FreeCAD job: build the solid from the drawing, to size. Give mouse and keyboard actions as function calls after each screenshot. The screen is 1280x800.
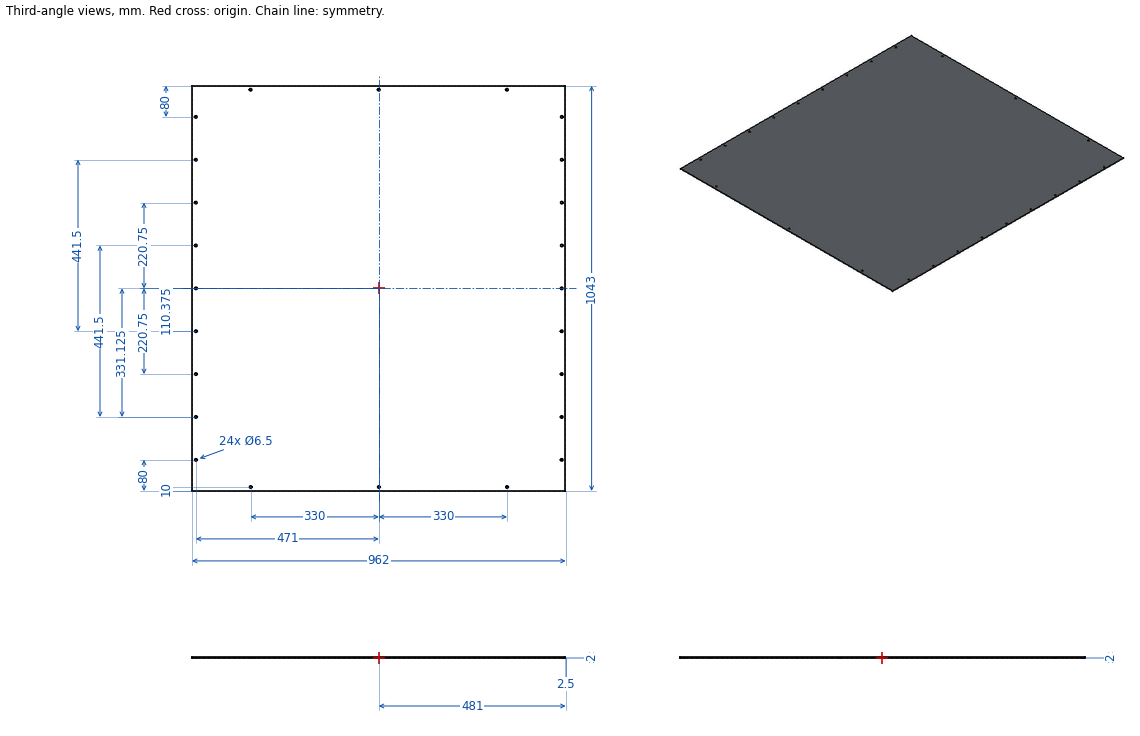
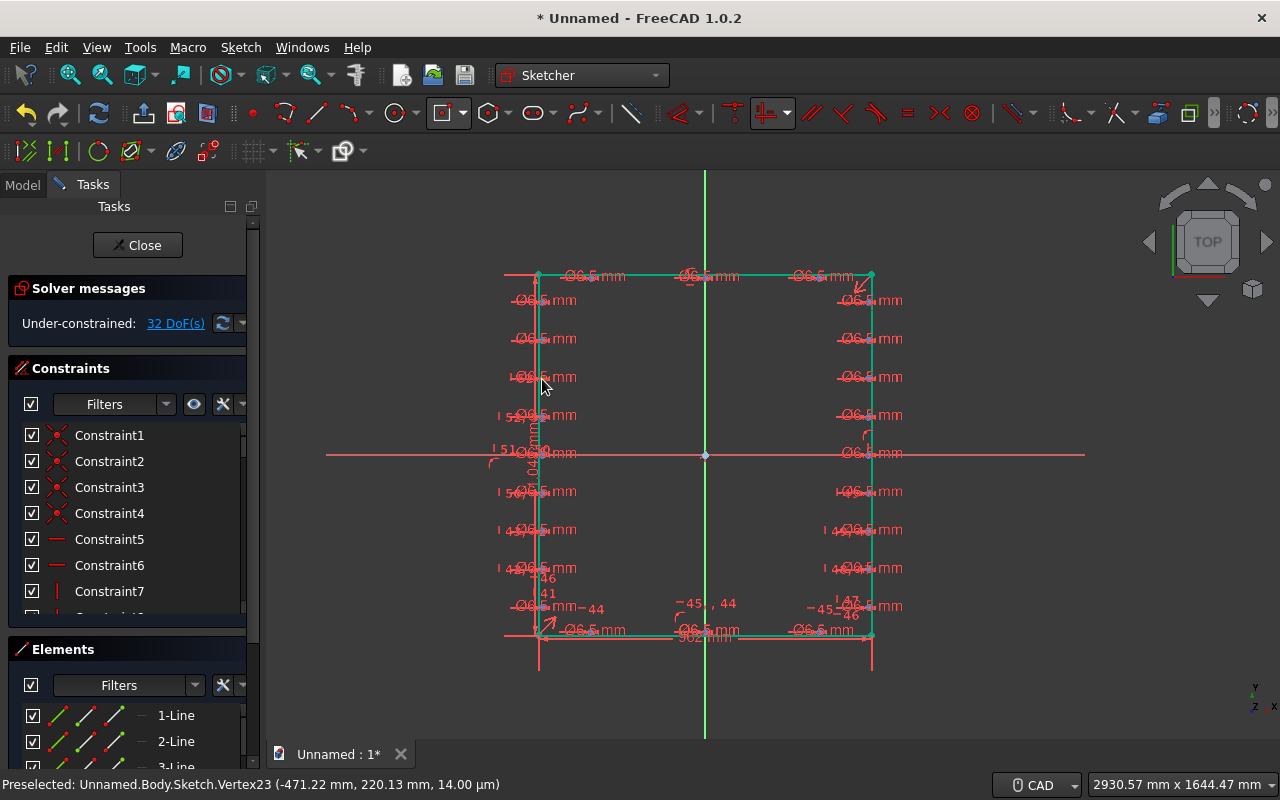
click(542, 341)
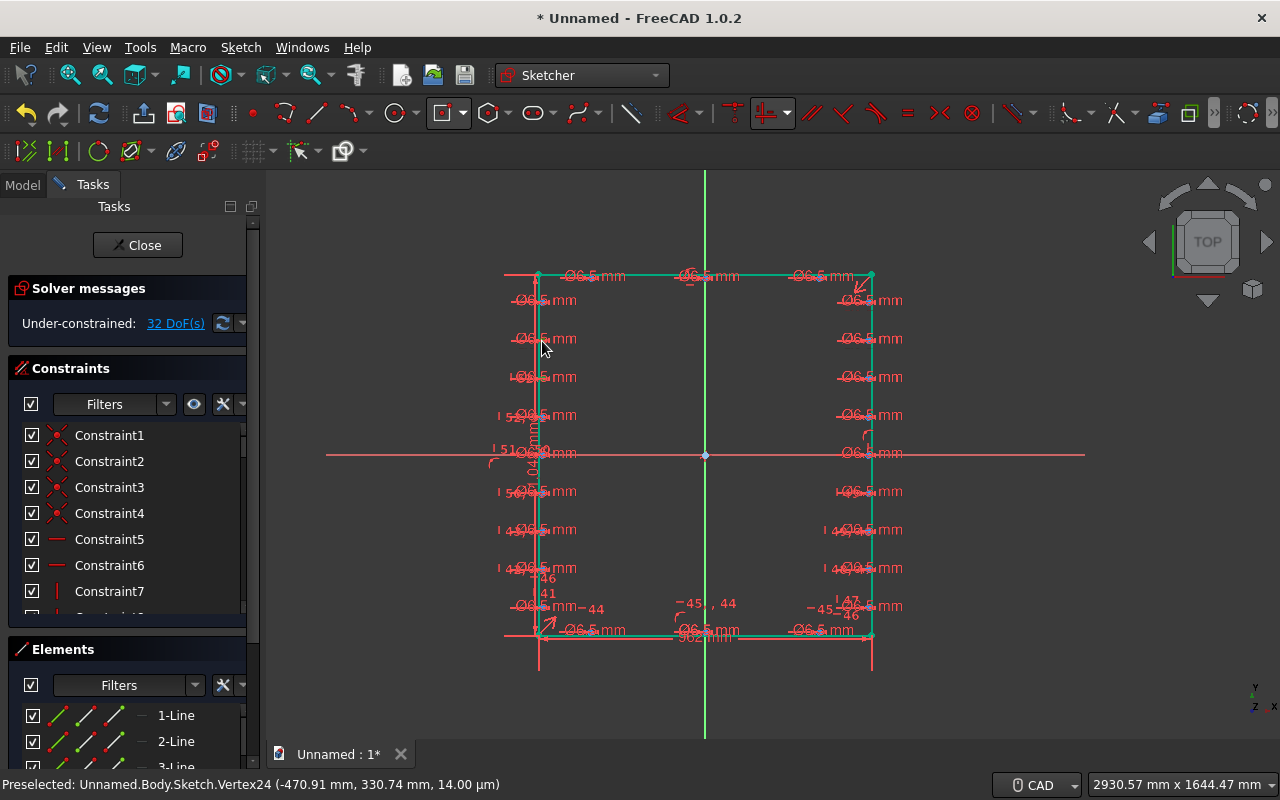
key(v)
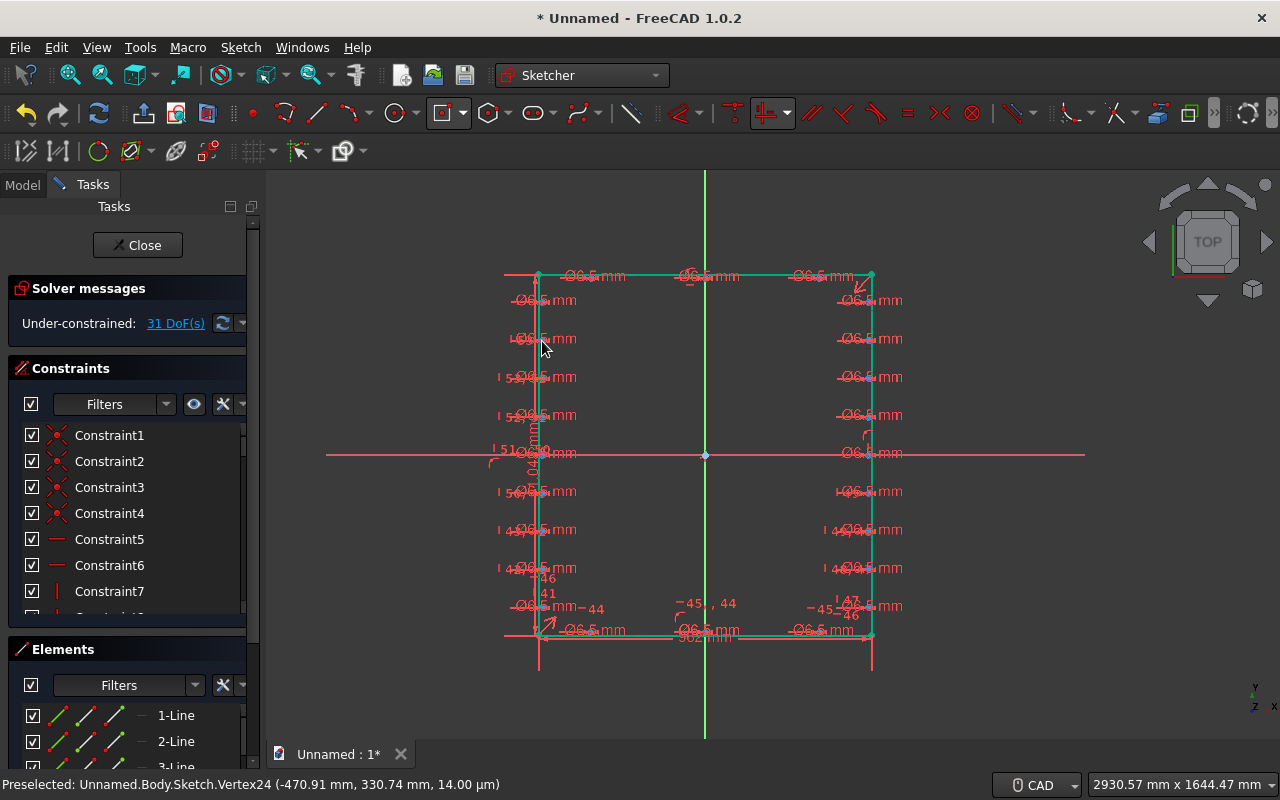
click(542, 341)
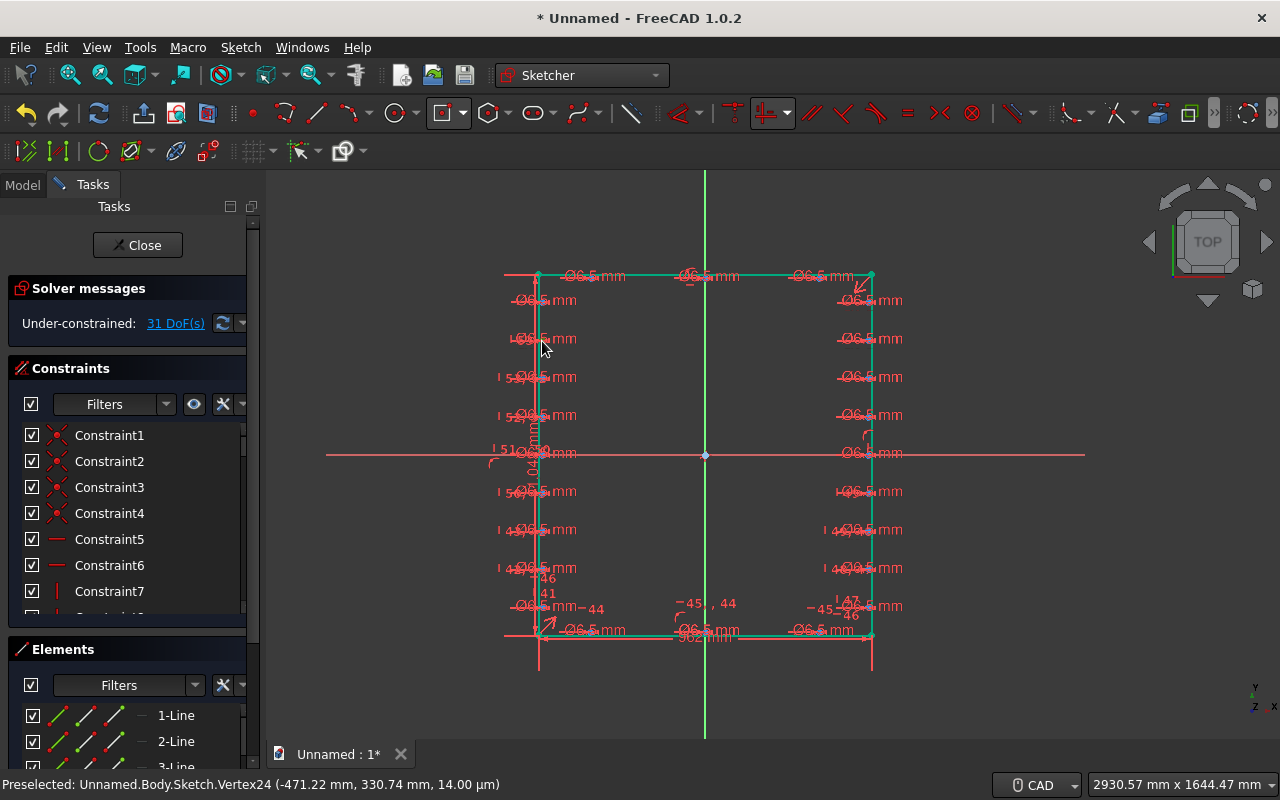
click(542, 302)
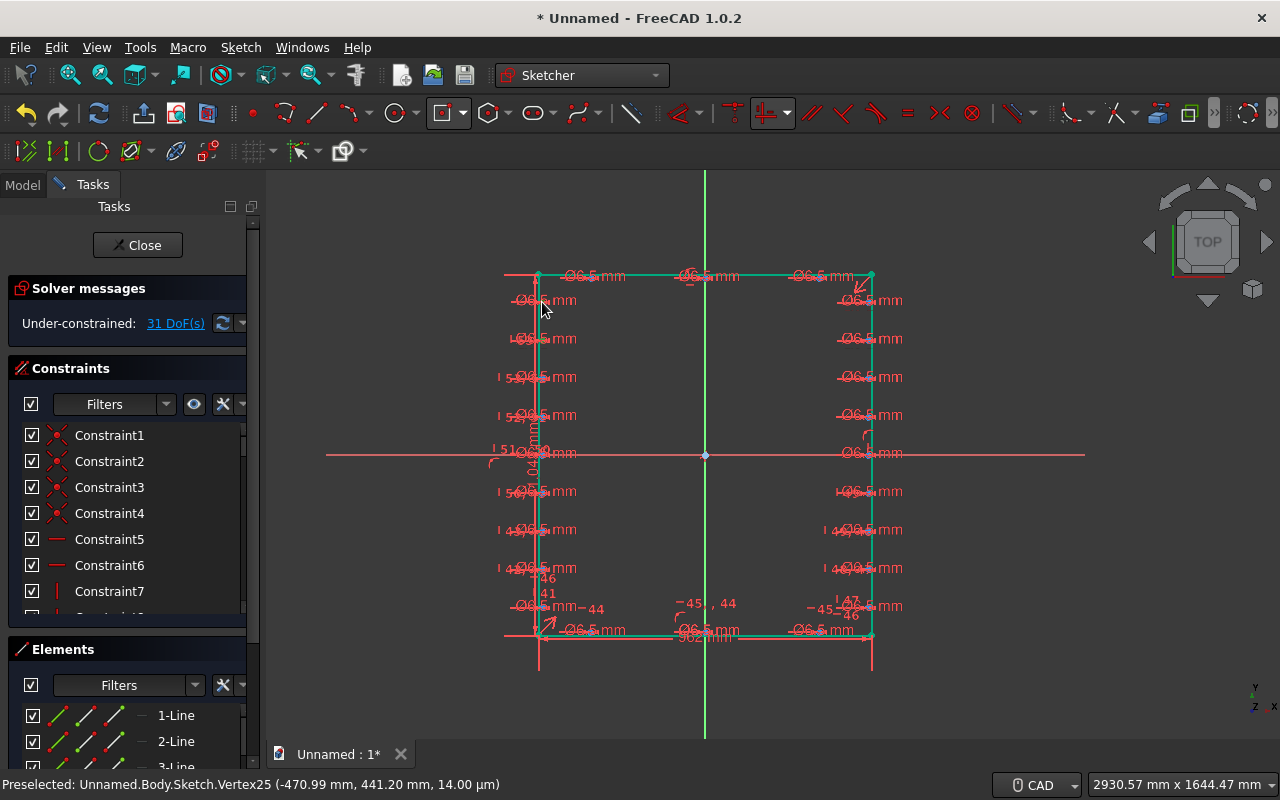
key(v)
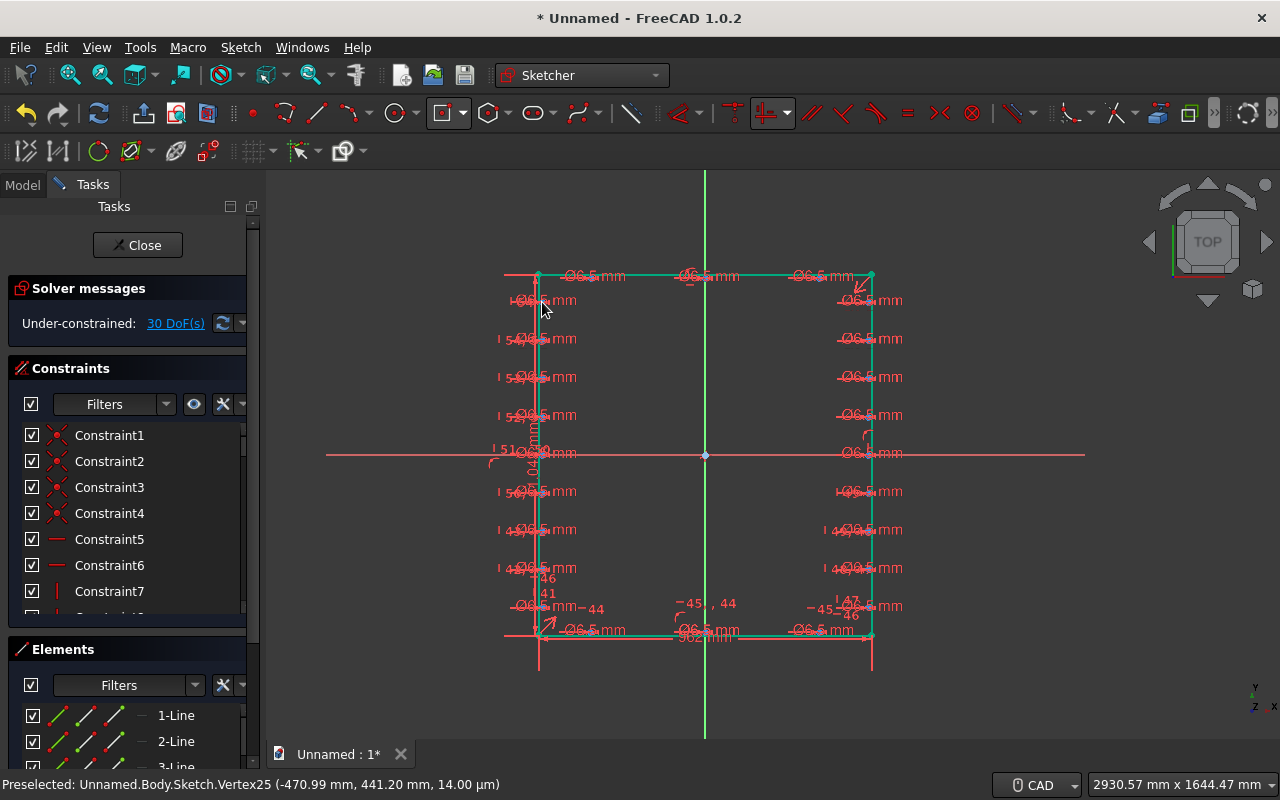
click(868, 493)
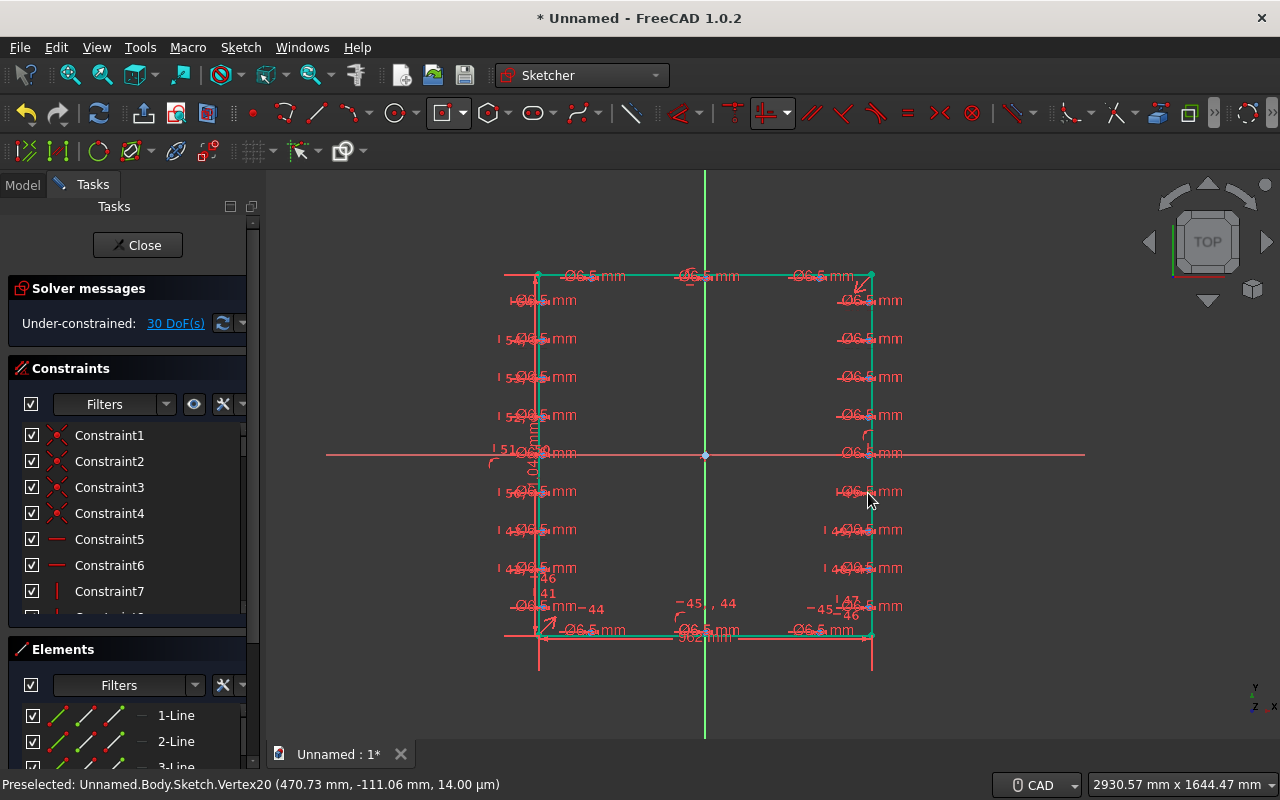
click(868, 455)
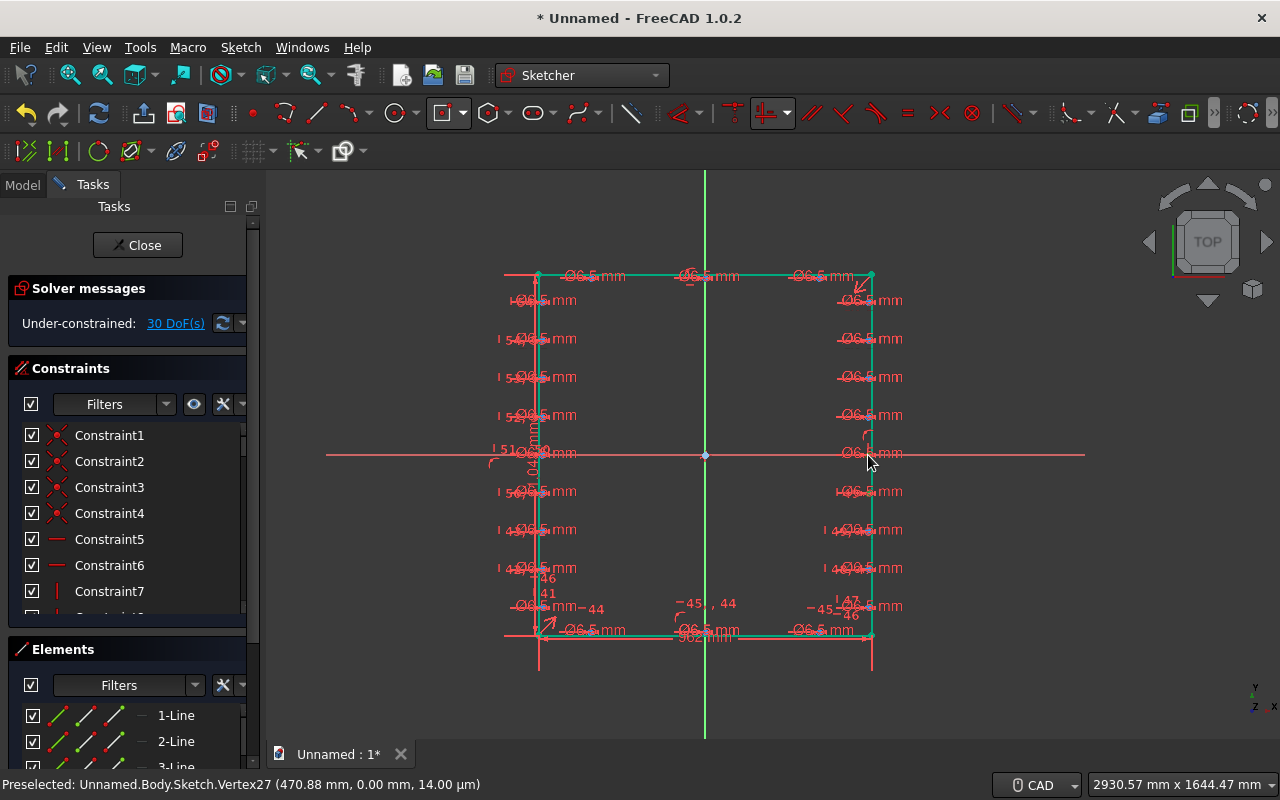
click(790, 114)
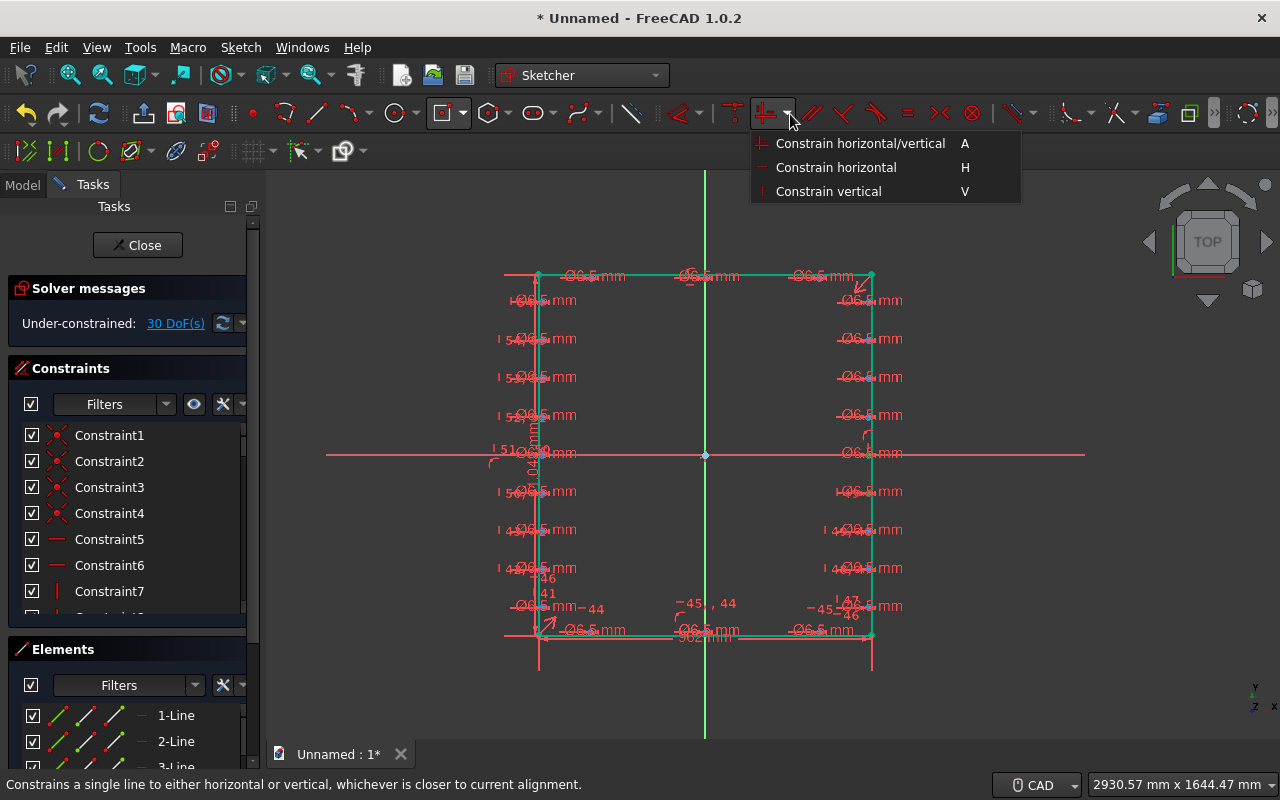
click(886, 191)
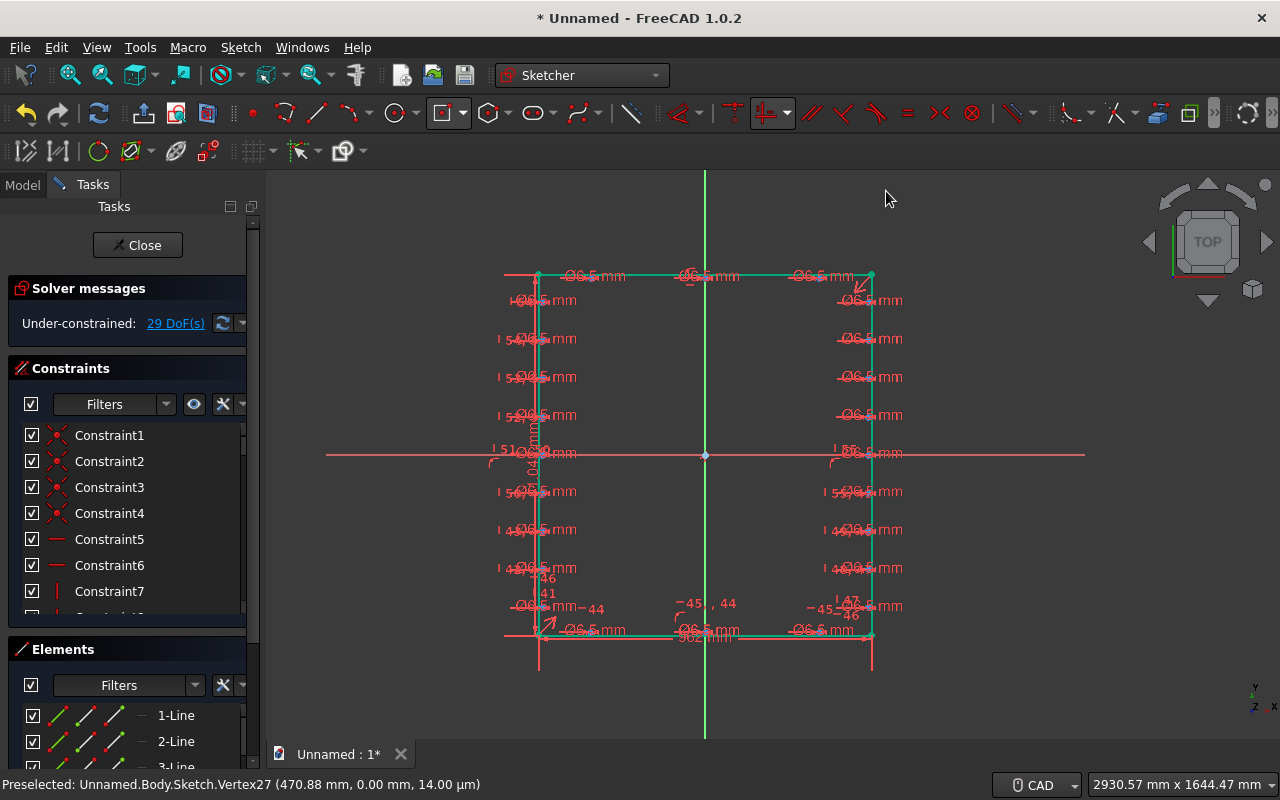
click(868, 455)